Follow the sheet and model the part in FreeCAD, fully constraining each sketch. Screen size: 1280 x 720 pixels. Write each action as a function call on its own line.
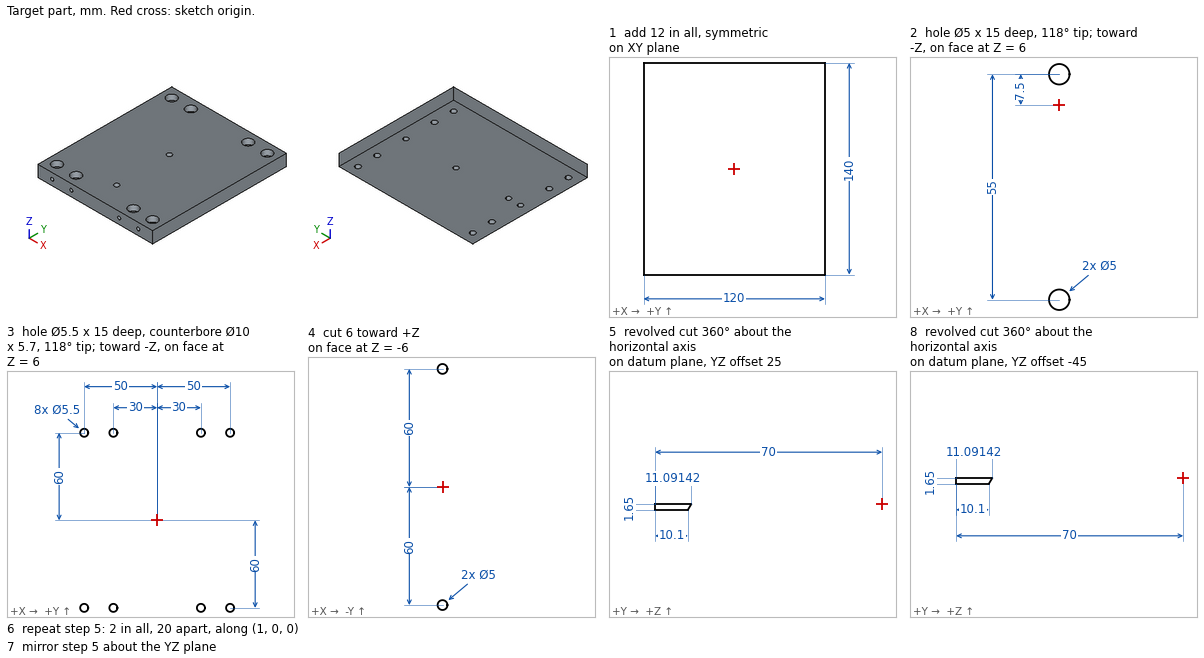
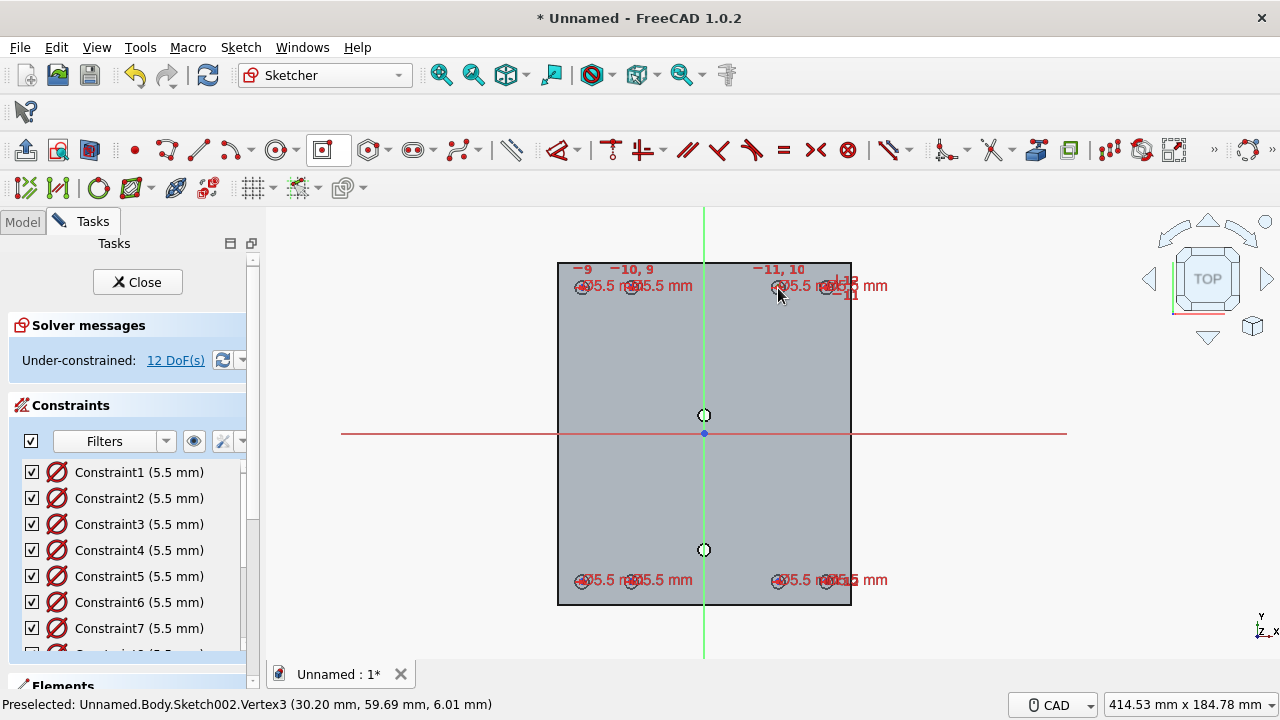
click(778, 582)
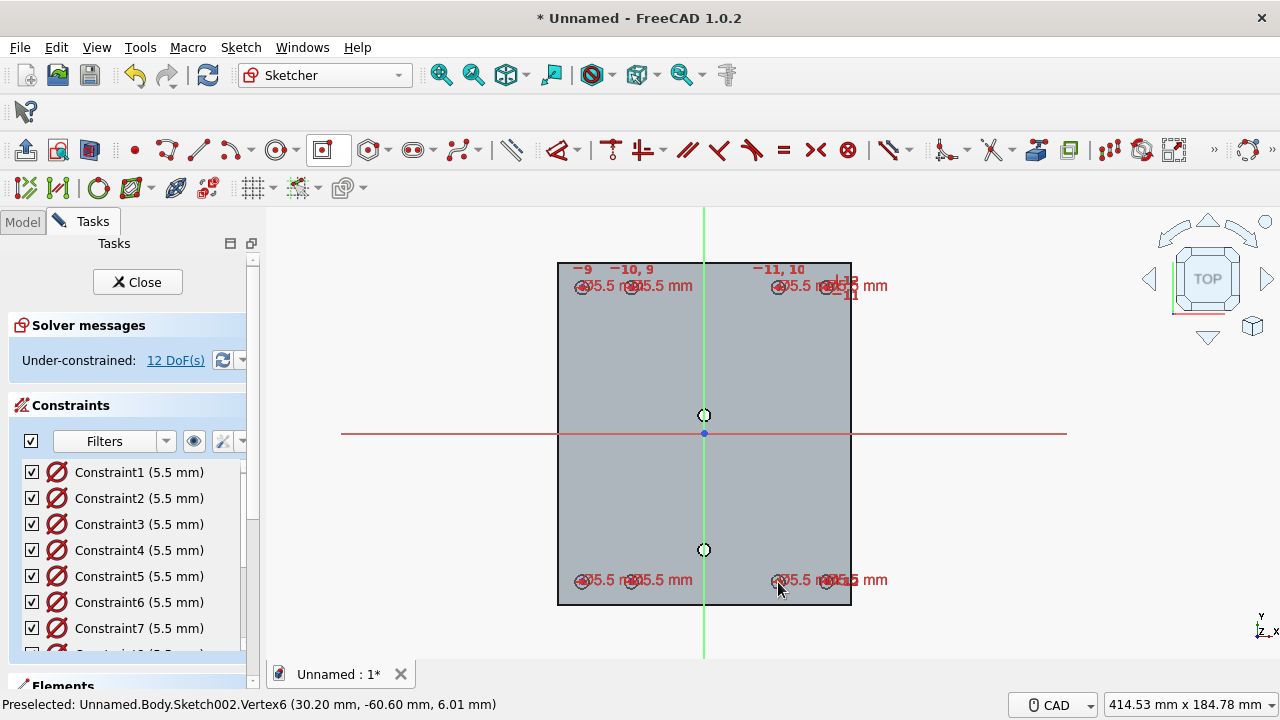
key(v)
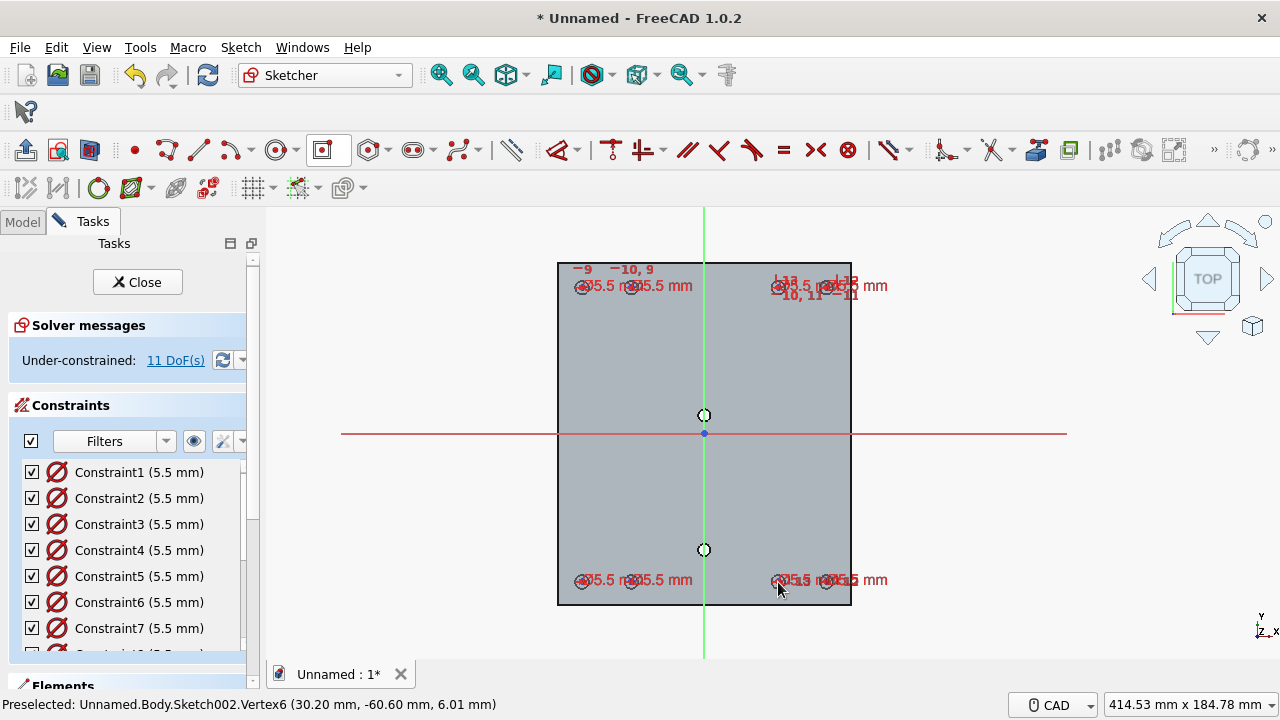
click(826, 582)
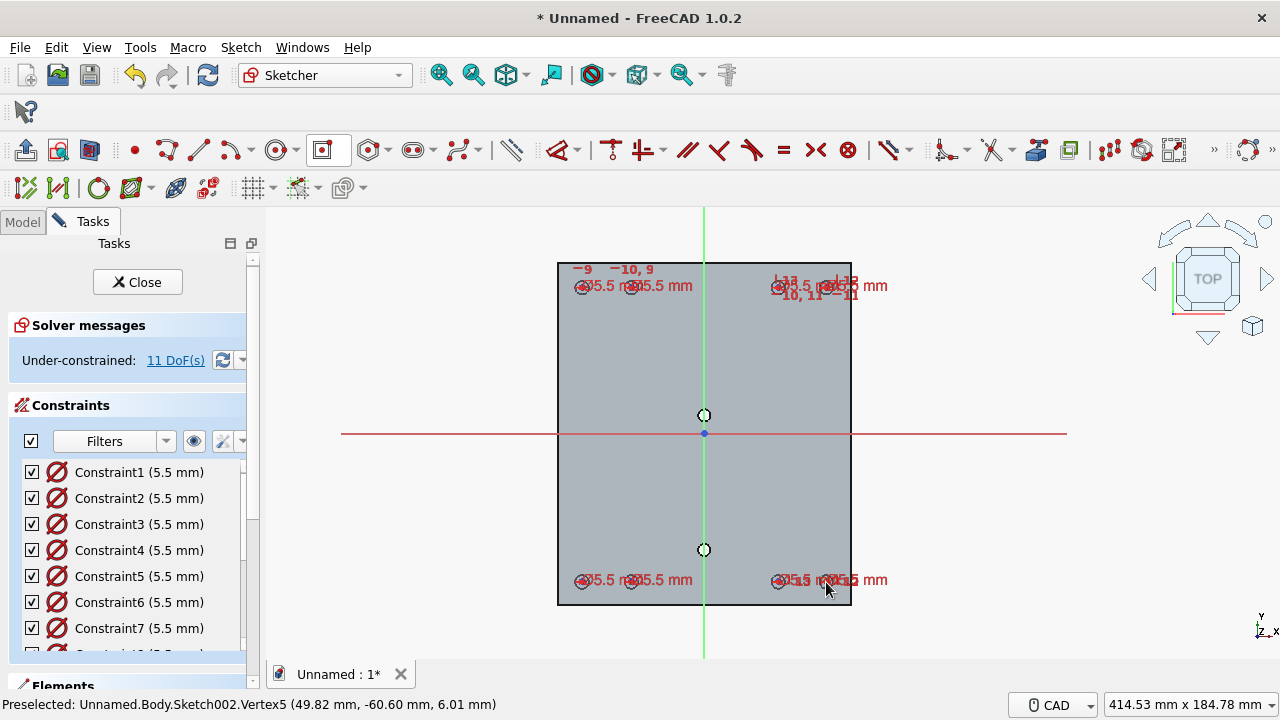
click(778, 582)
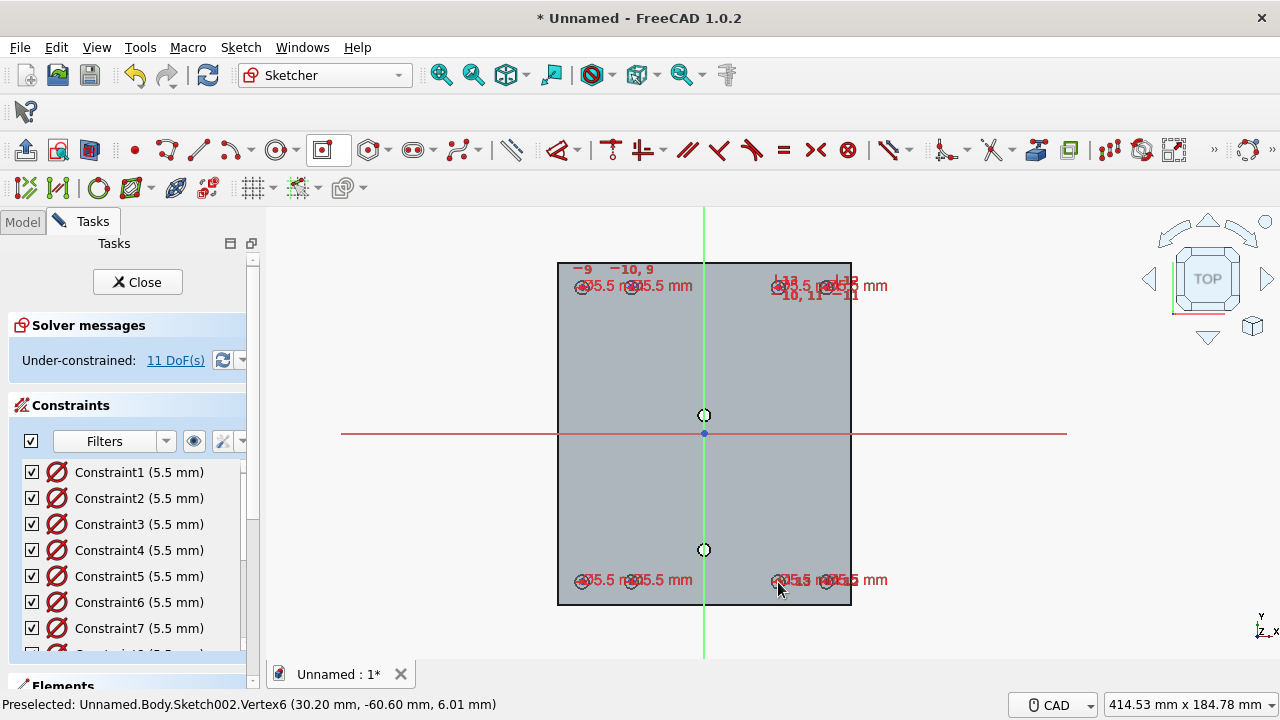
key(h)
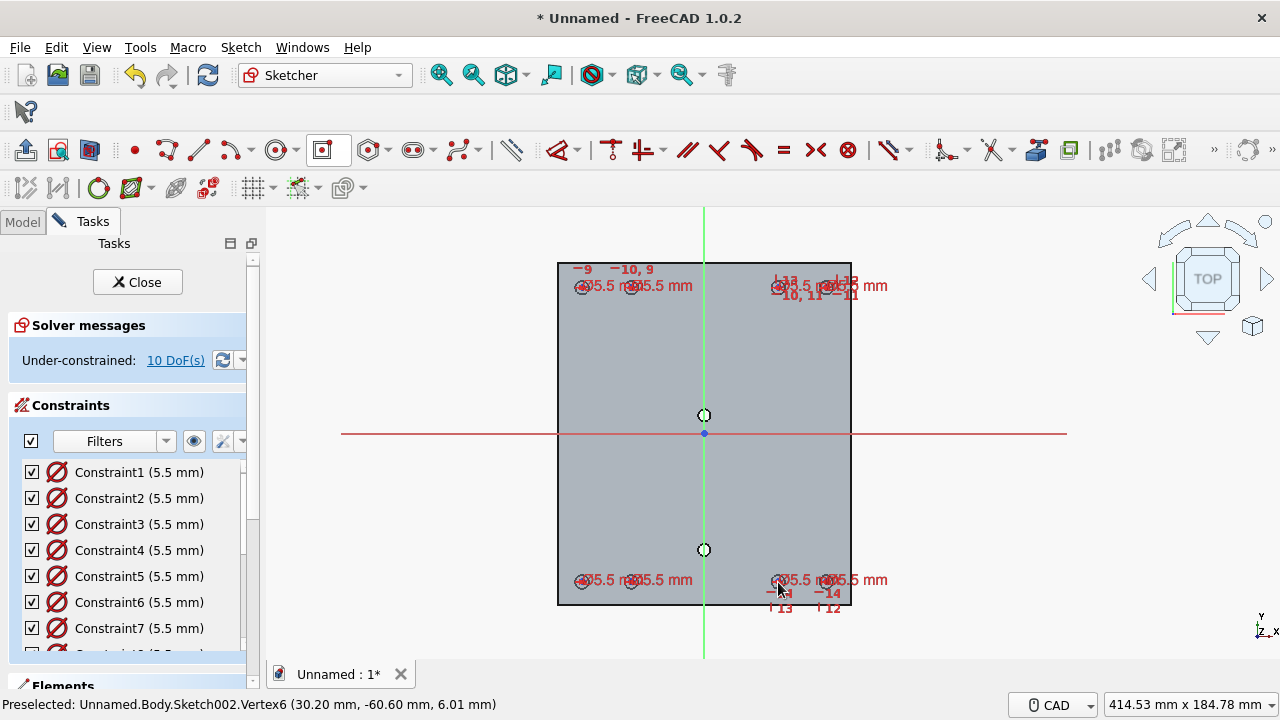
click(631, 288)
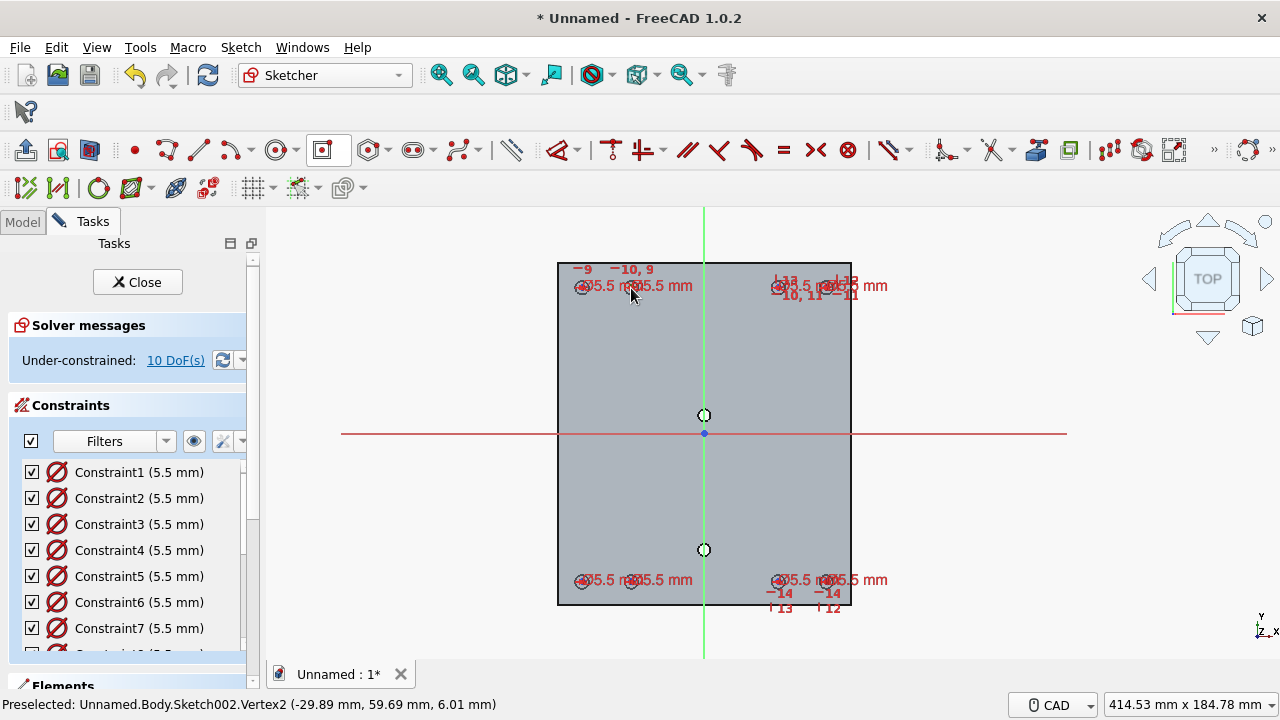
click(631, 582)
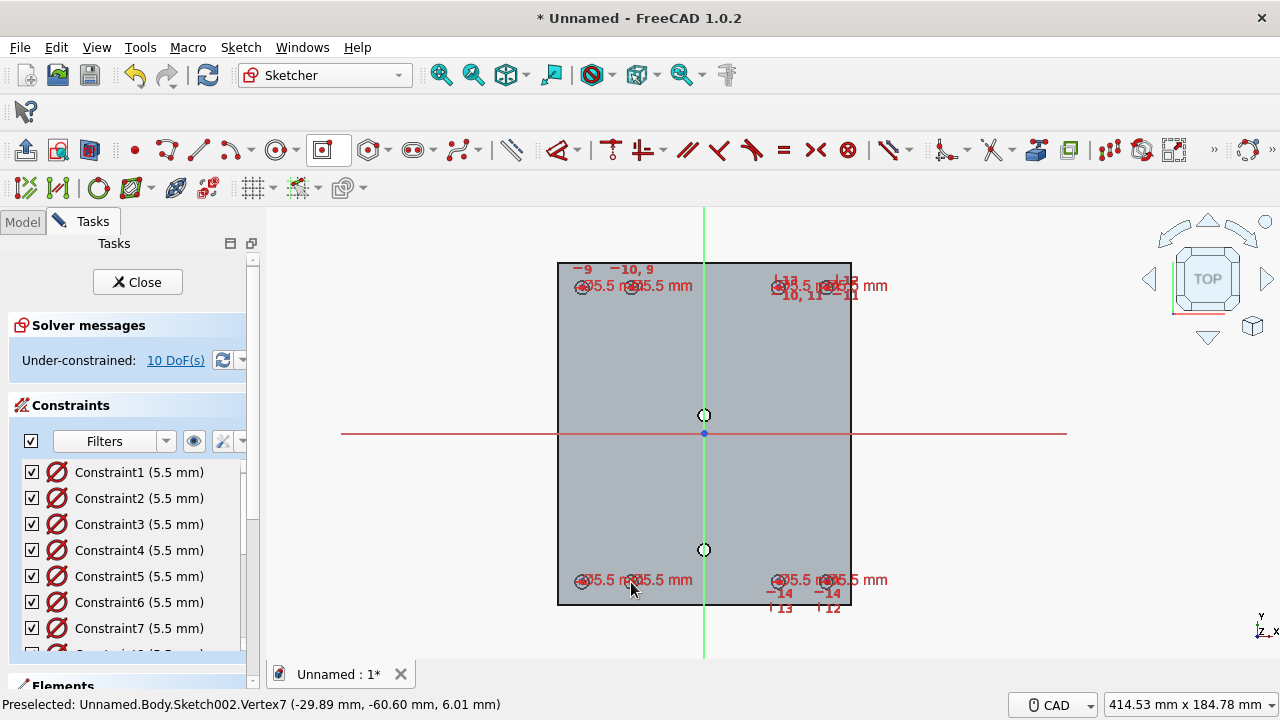
key(v)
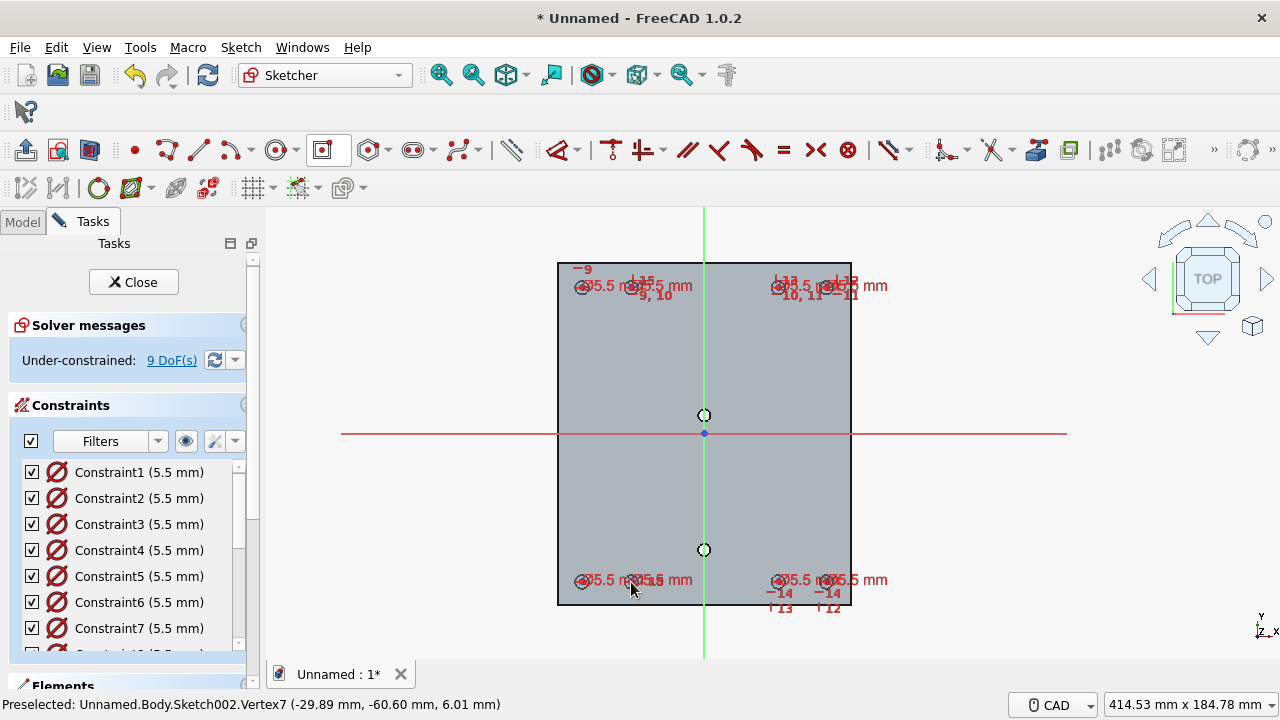
click(778, 582)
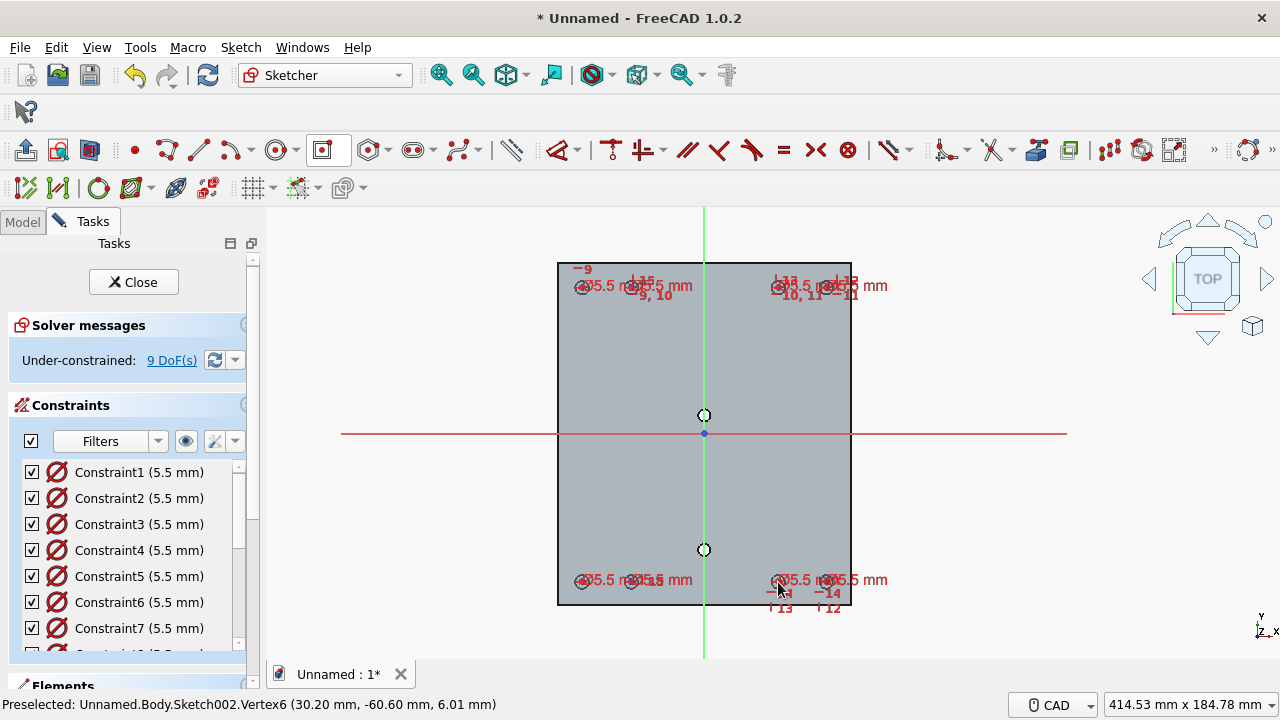
click(631, 582)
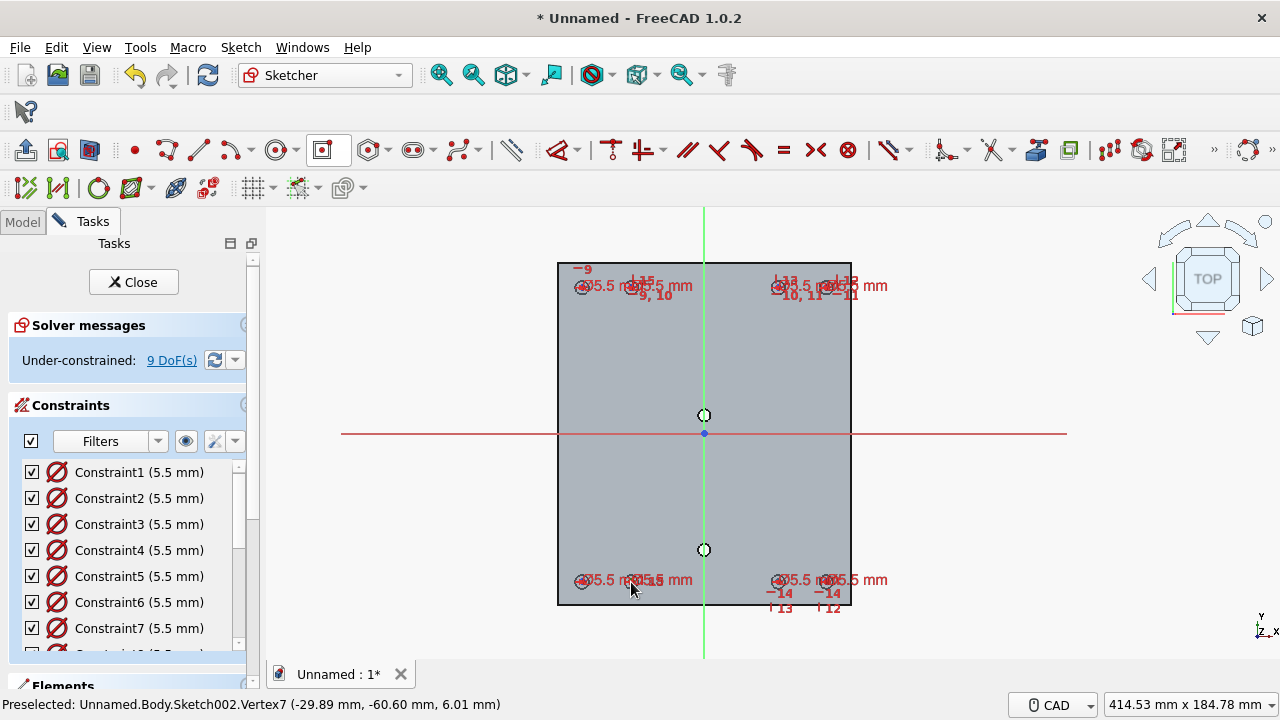
key(h)